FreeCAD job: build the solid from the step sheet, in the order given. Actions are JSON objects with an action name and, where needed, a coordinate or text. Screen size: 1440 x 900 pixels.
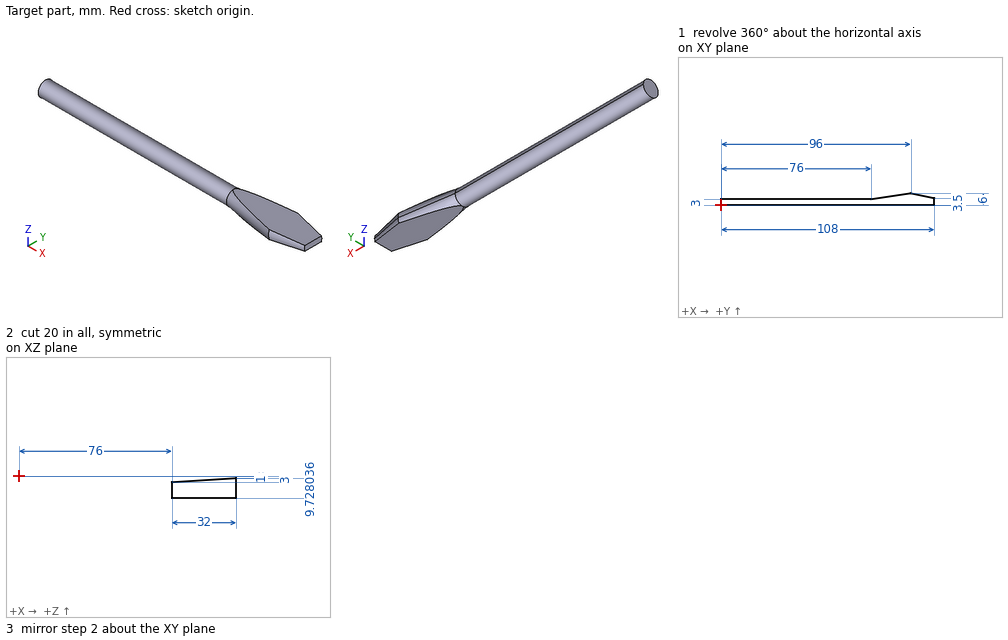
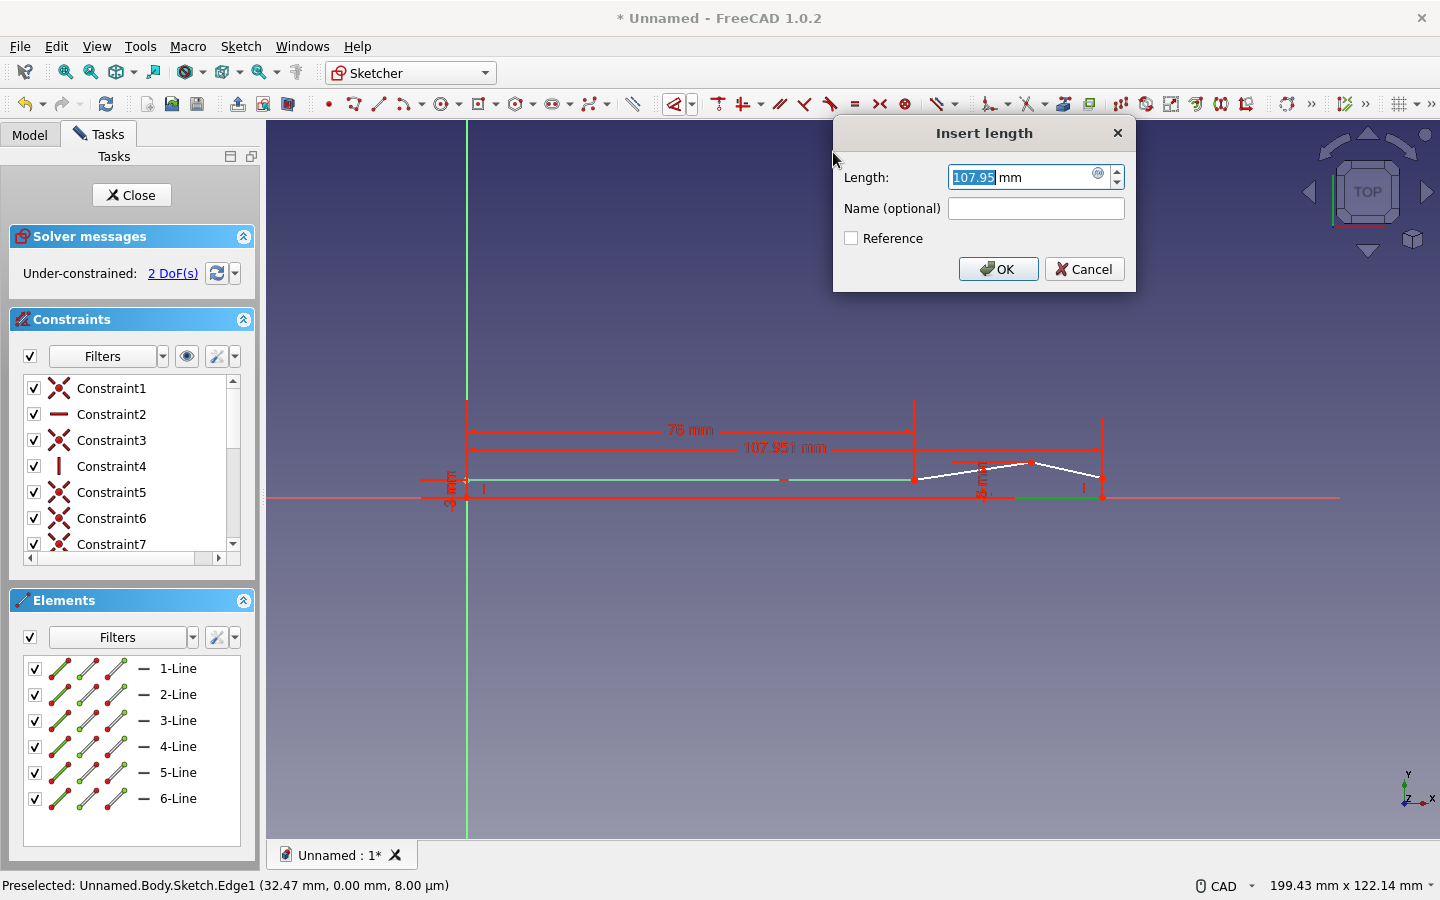
{"action": "type", "text": "108"}
{"action": "key", "text": "Return"}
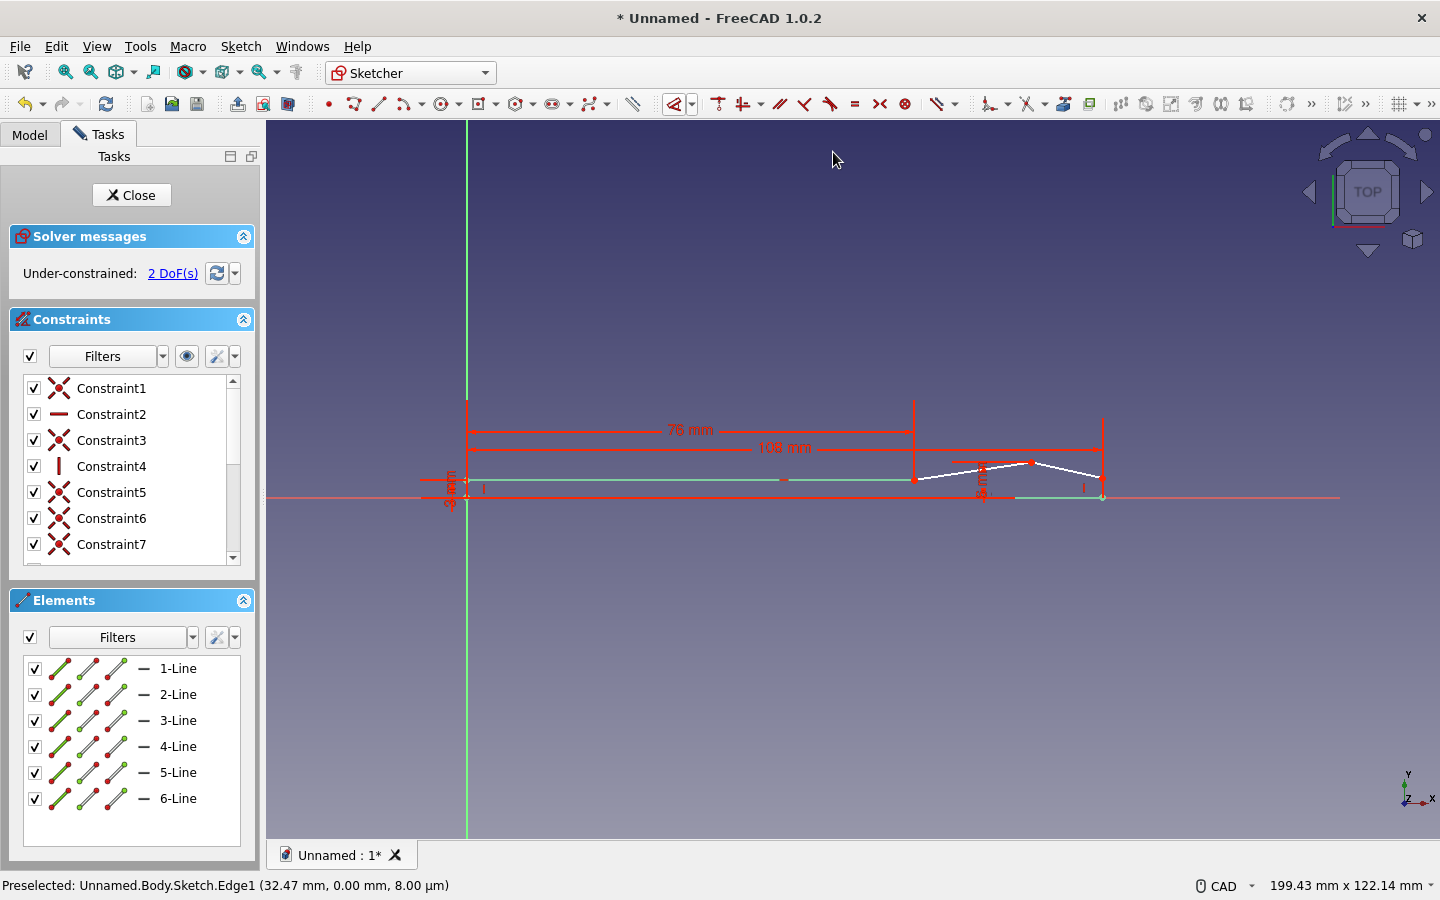
{"action": "scroll", "coordinate": [1103, 488], "scroll_direction": "up", "scroll_amount": 4}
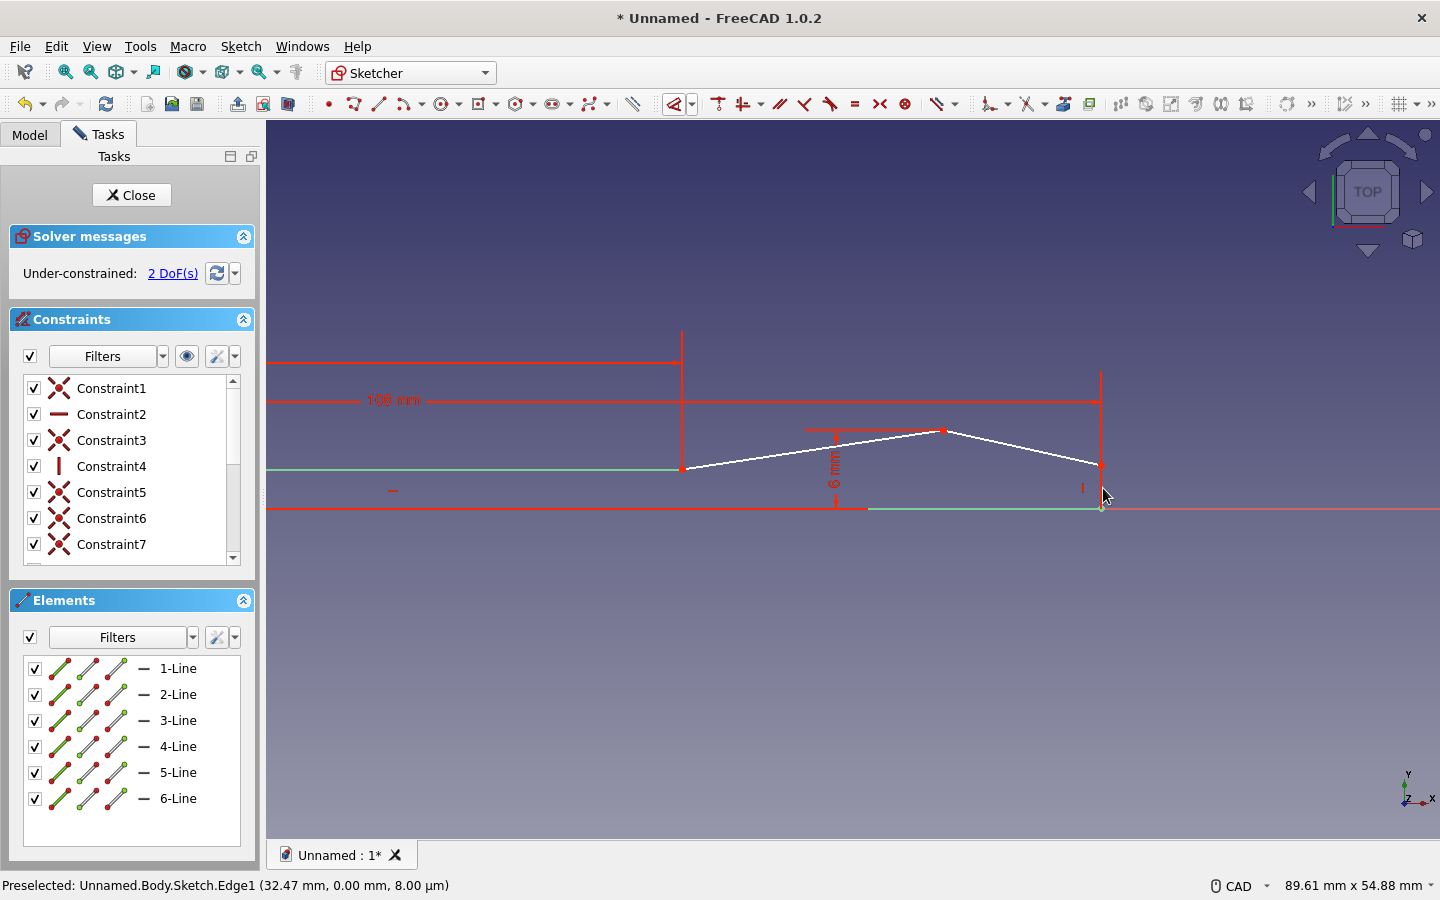
{"action": "left_click", "coordinate": [1101, 487]}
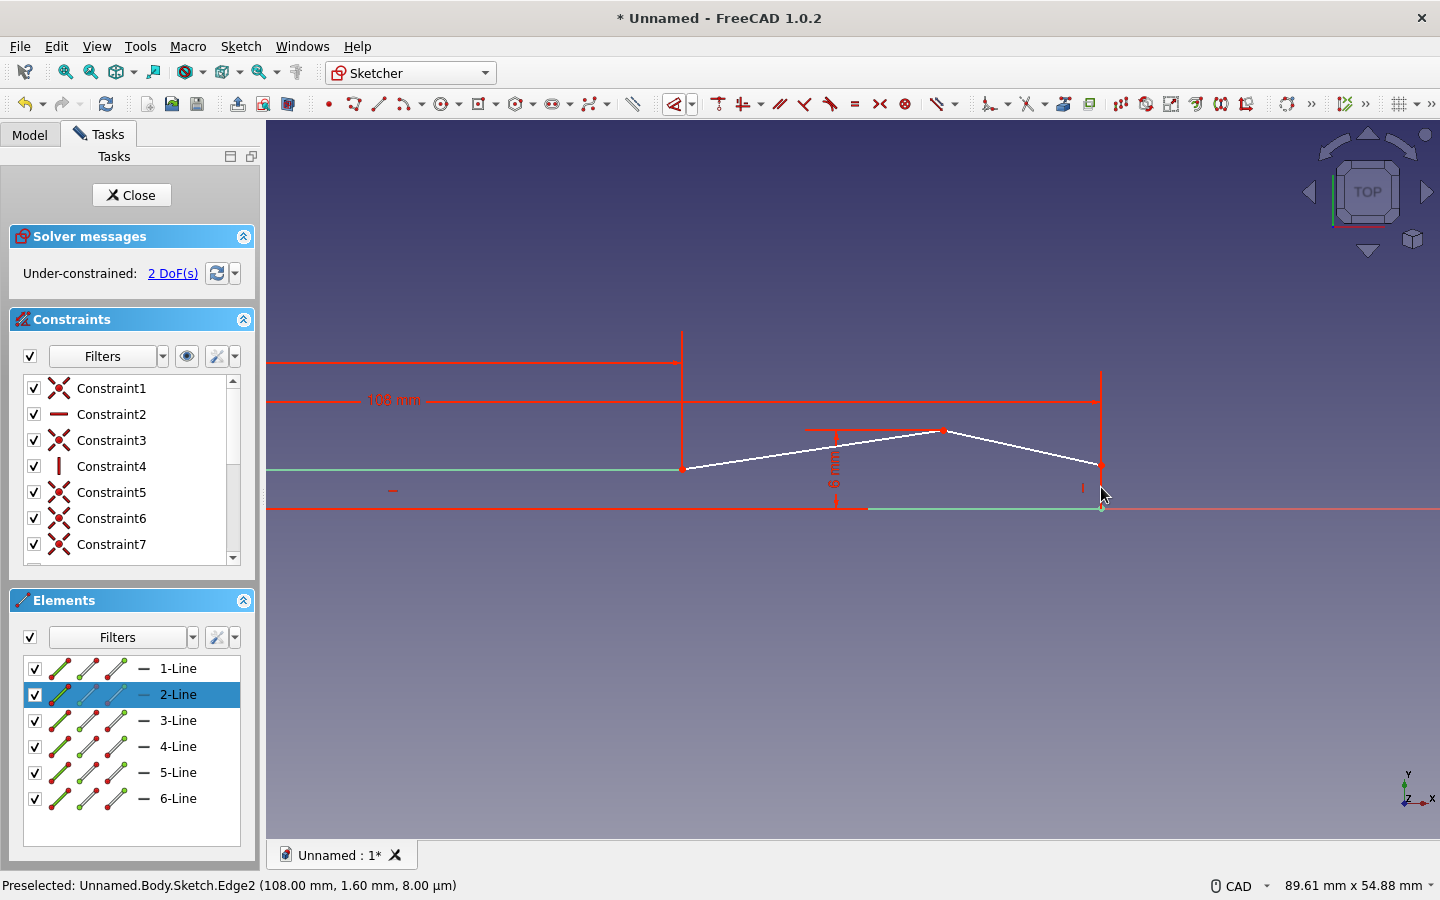
{"action": "left_click", "coordinate": [692, 104]}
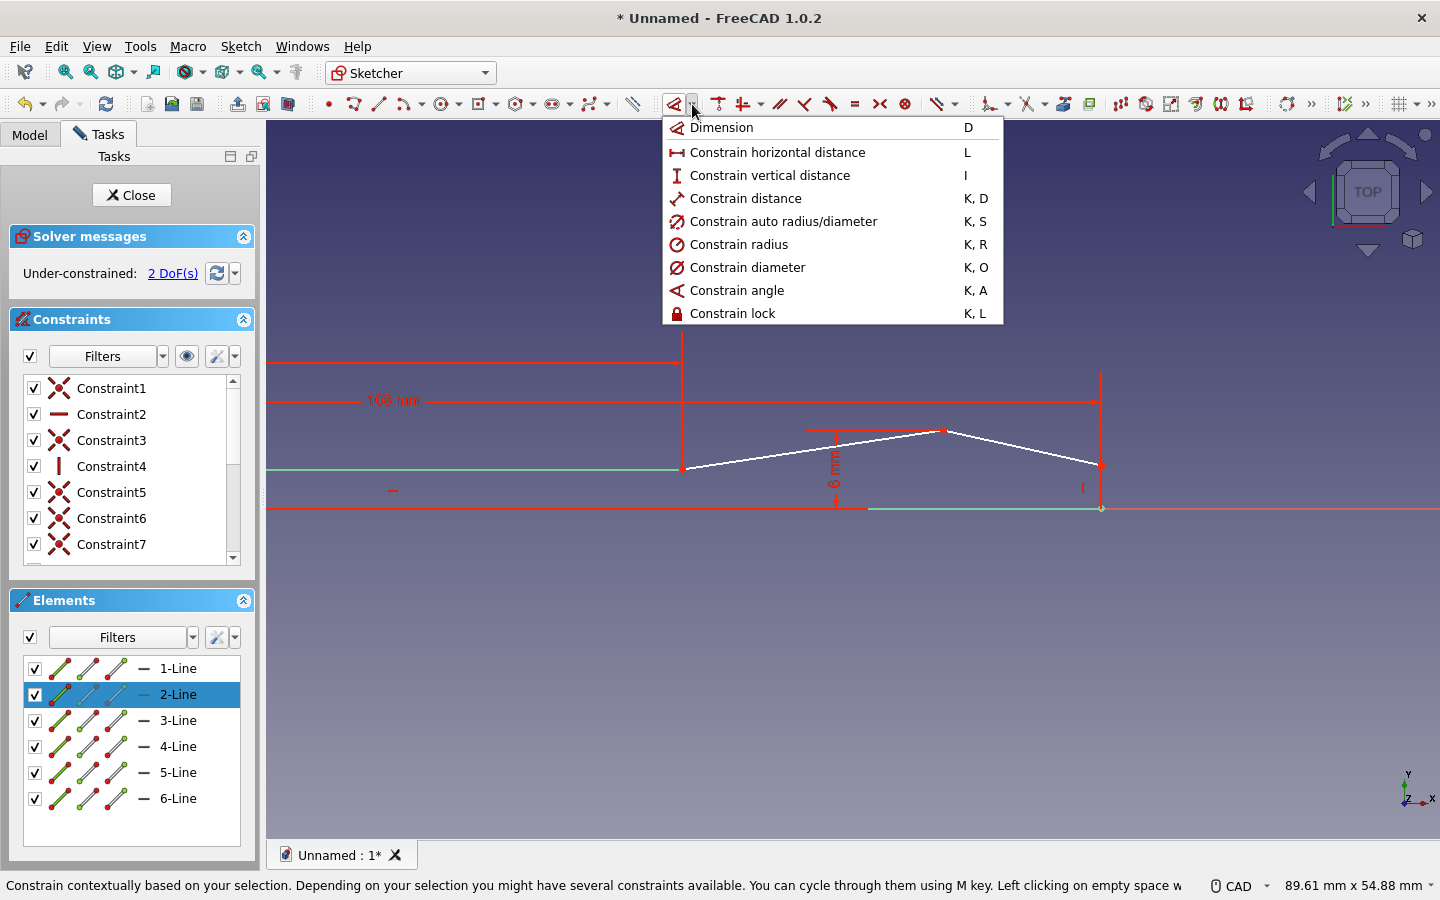
{"action": "left_click", "coordinate": [833, 176]}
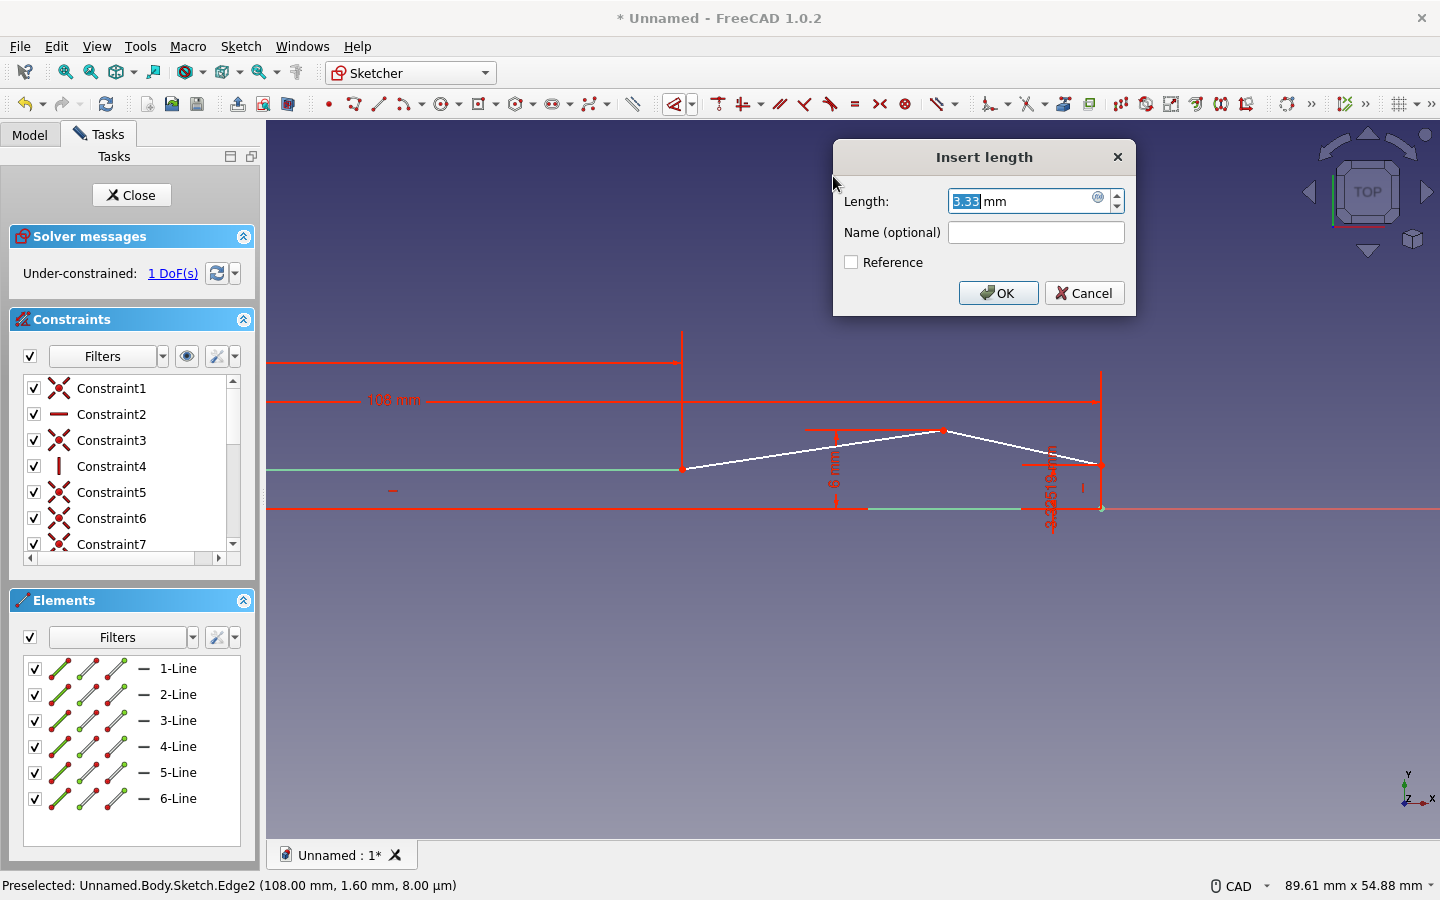
{"action": "type", "text": "3.5"}
{"action": "key", "text": "Return"}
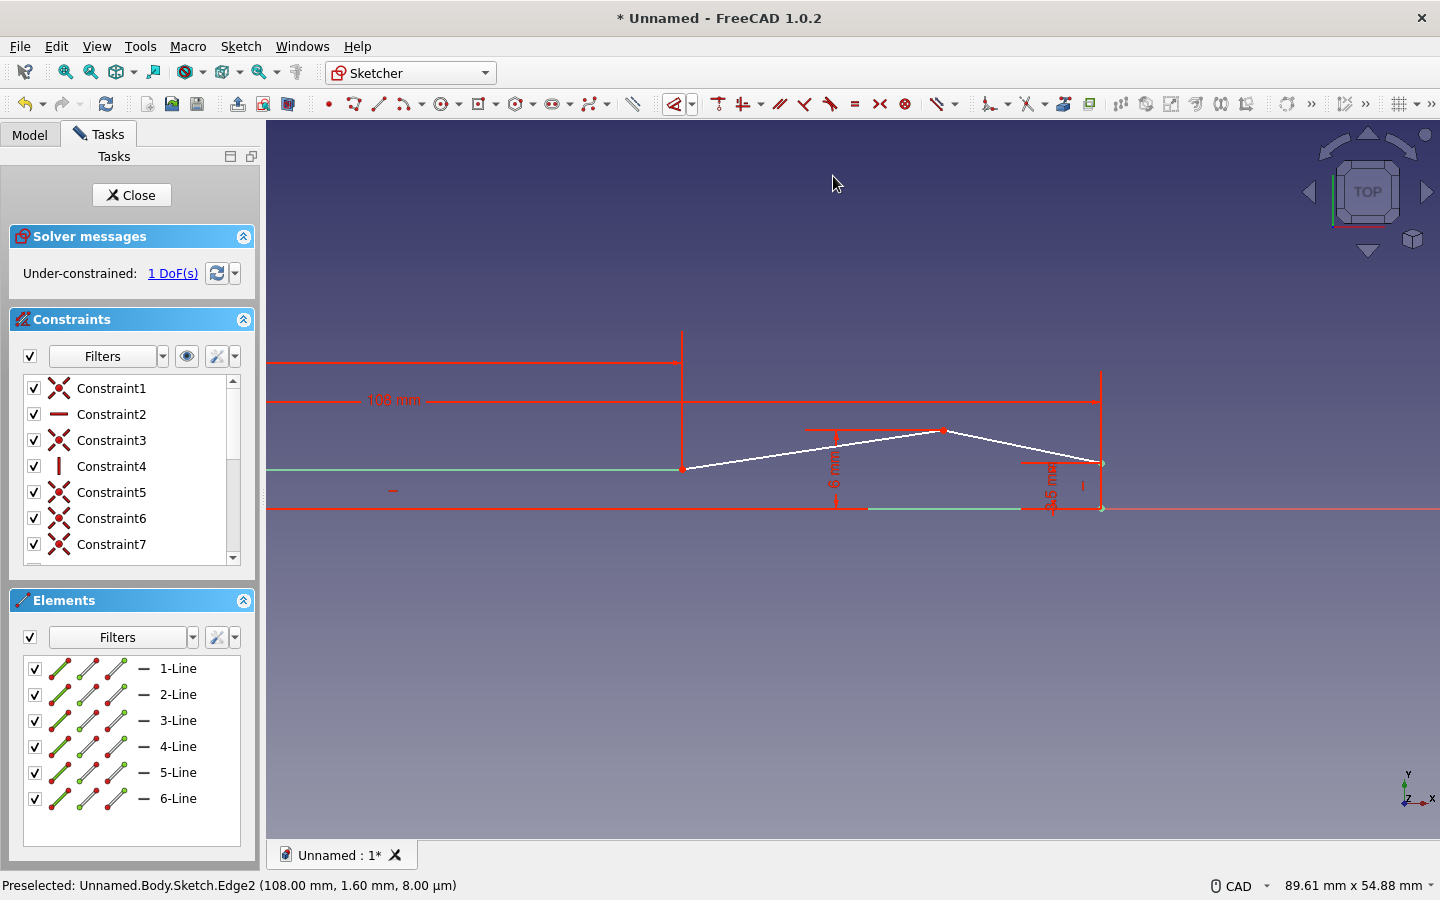
{"action": "left_click", "coordinate": [943, 430]}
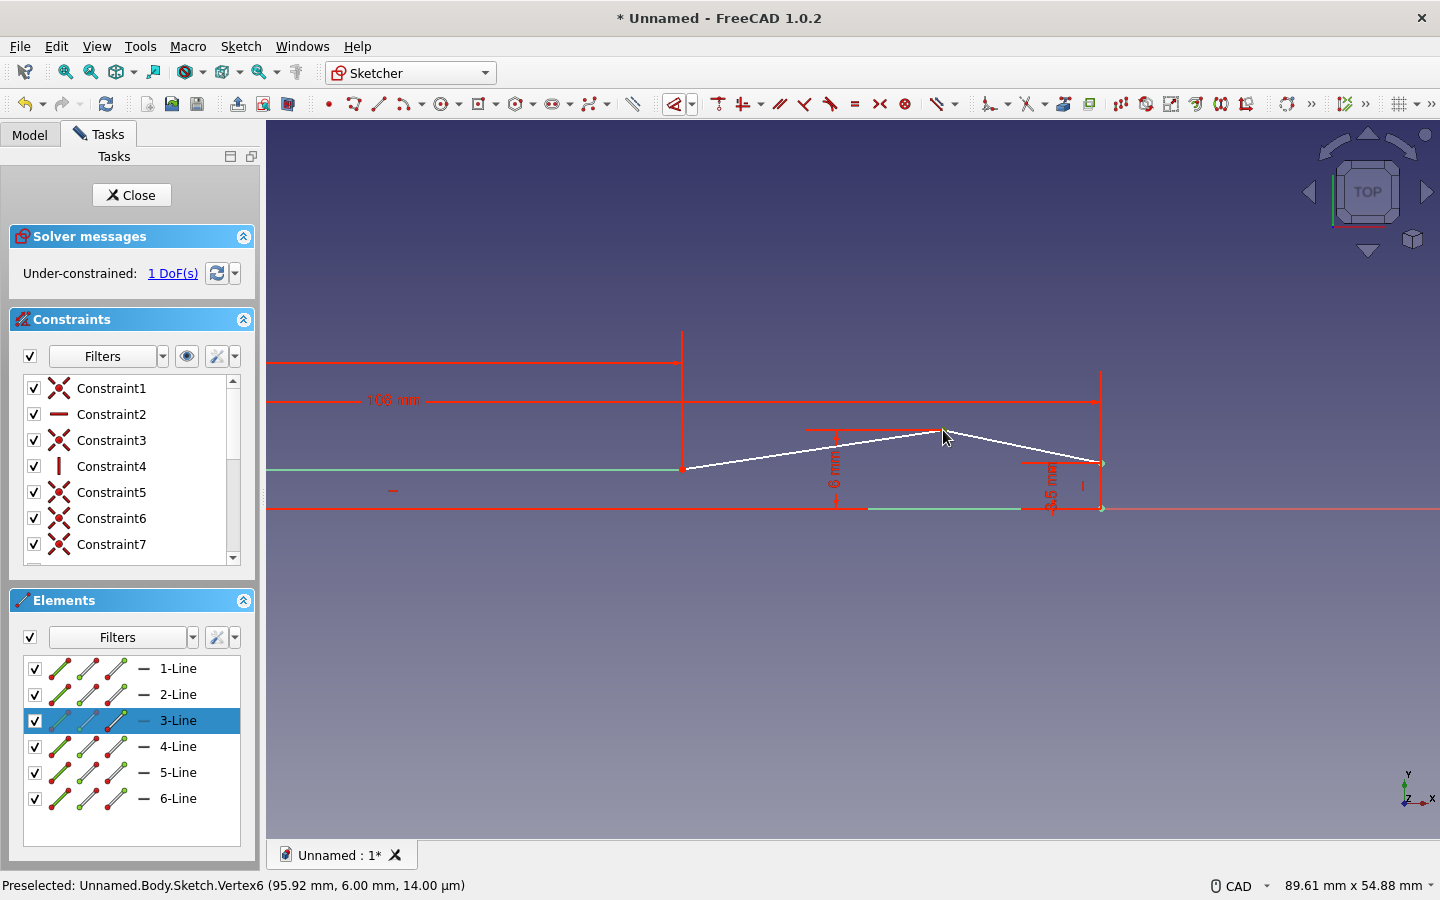
{"action": "key", "text": "l"}